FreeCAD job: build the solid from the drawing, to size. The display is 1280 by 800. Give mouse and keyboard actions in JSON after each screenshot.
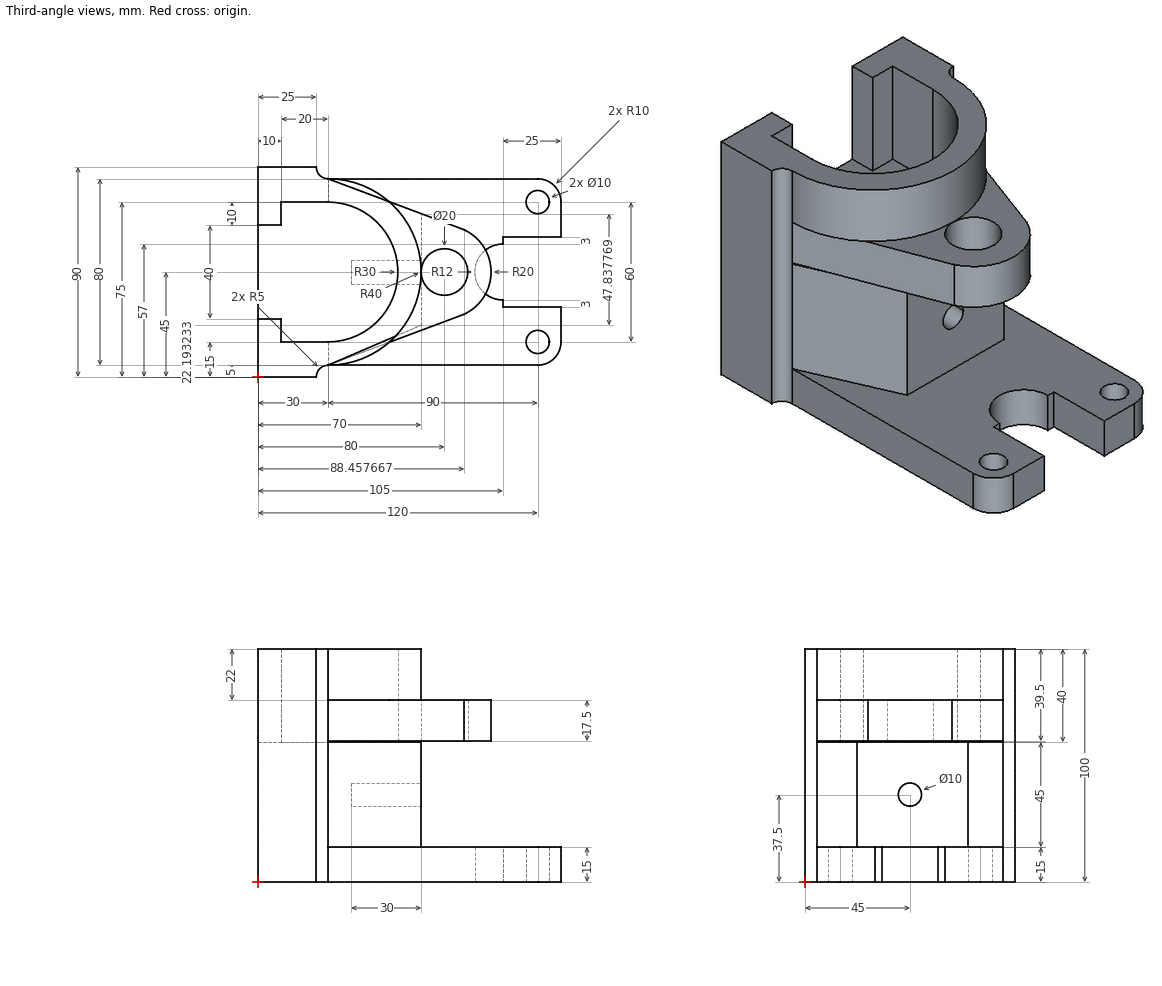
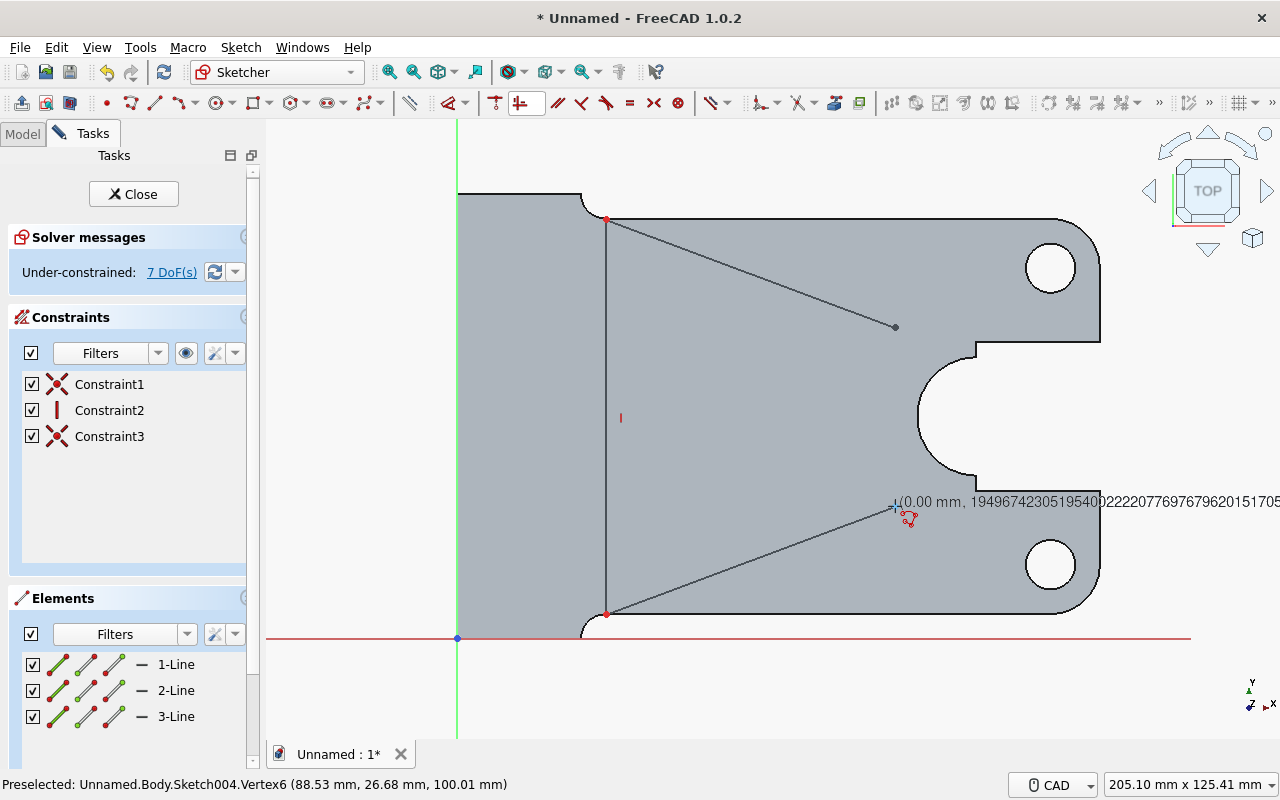
{"action": "left_click", "coordinate": [180, 104]}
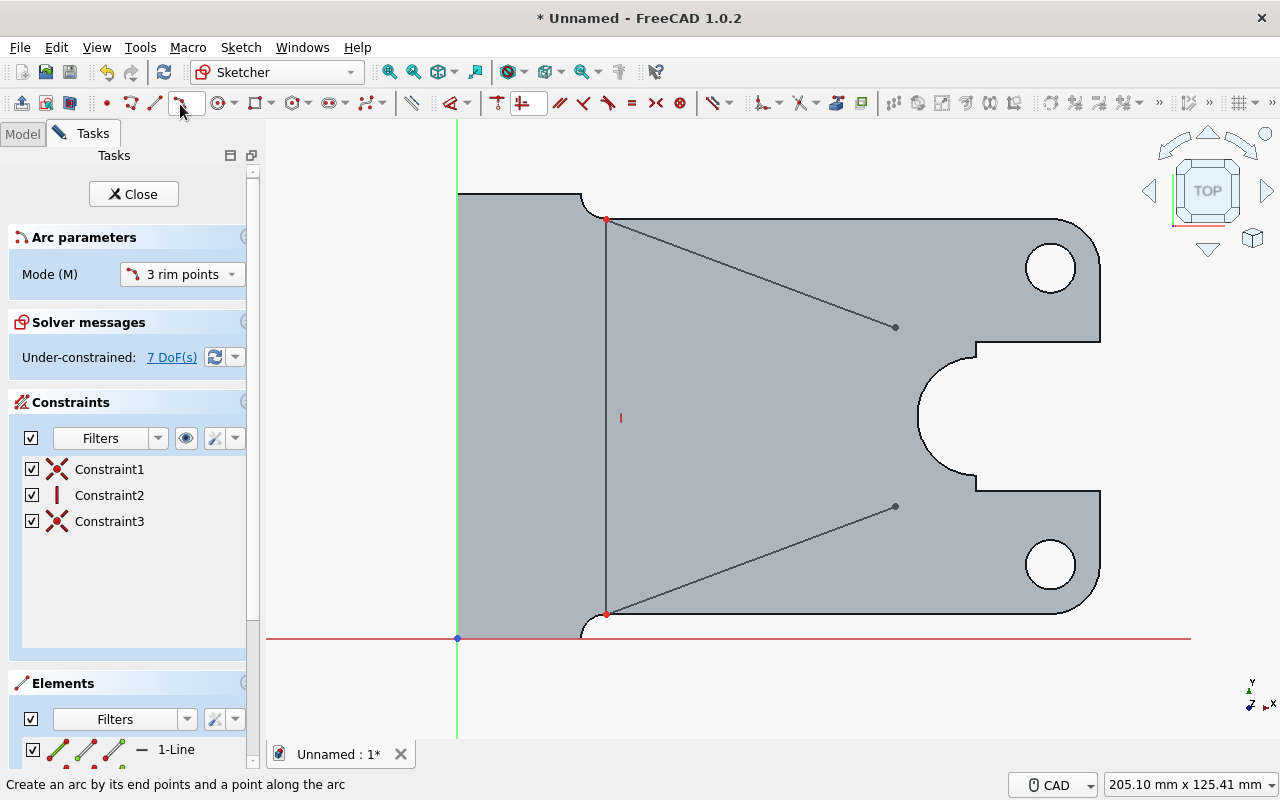
{"action": "left_click", "coordinate": [895, 507]}
{"action": "left_click", "coordinate": [895, 328]}
{"action": "left_click", "coordinate": [952, 416]}
{"action": "key", "text": "Escape"}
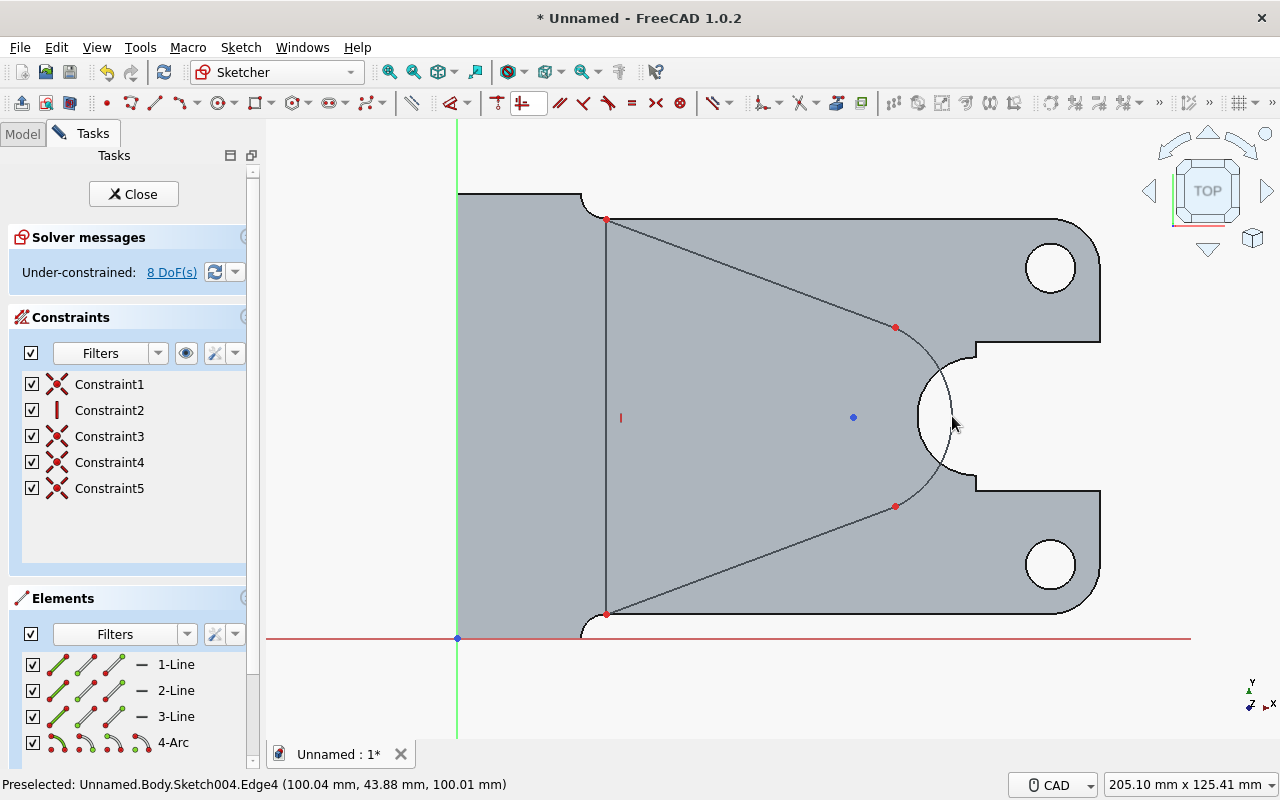
{"action": "key", "text": "d"}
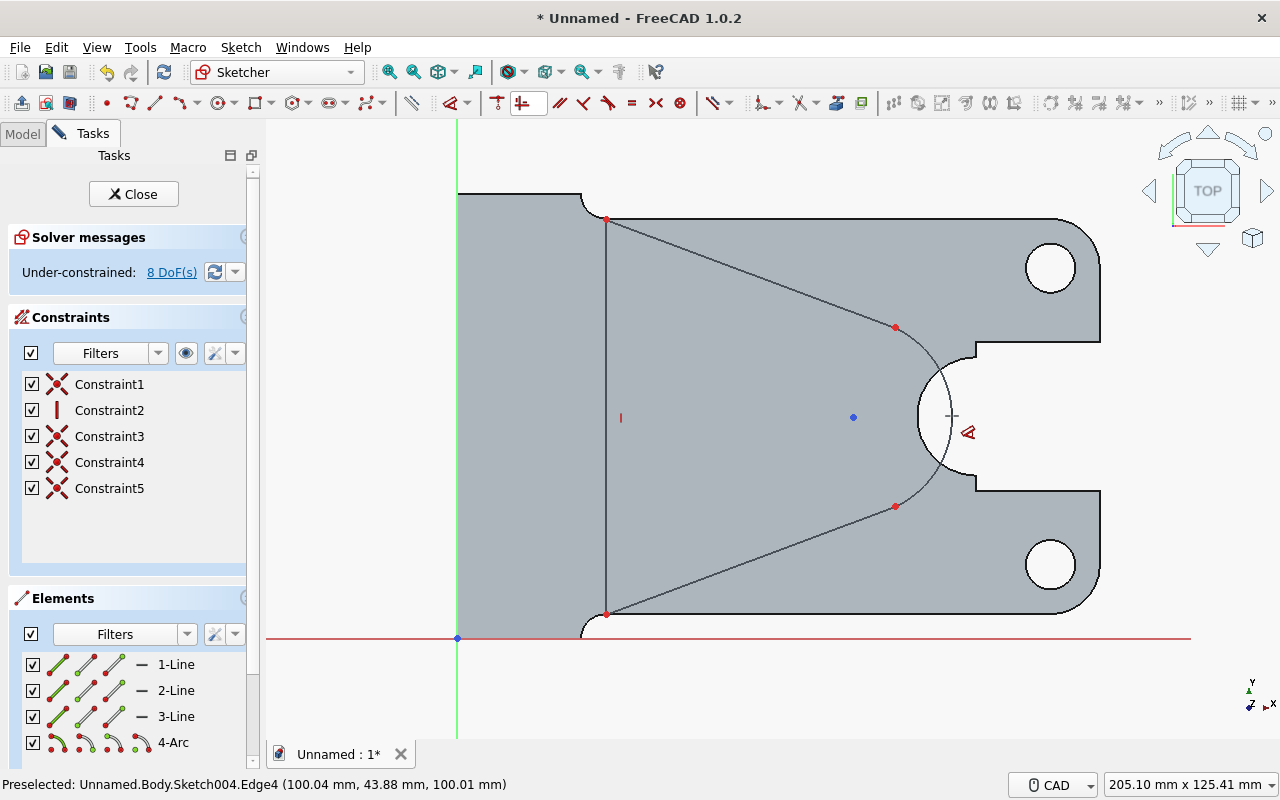
{"action": "left_click", "coordinate": [942, 461]}
{"action": "left_click", "coordinate": [971, 475]}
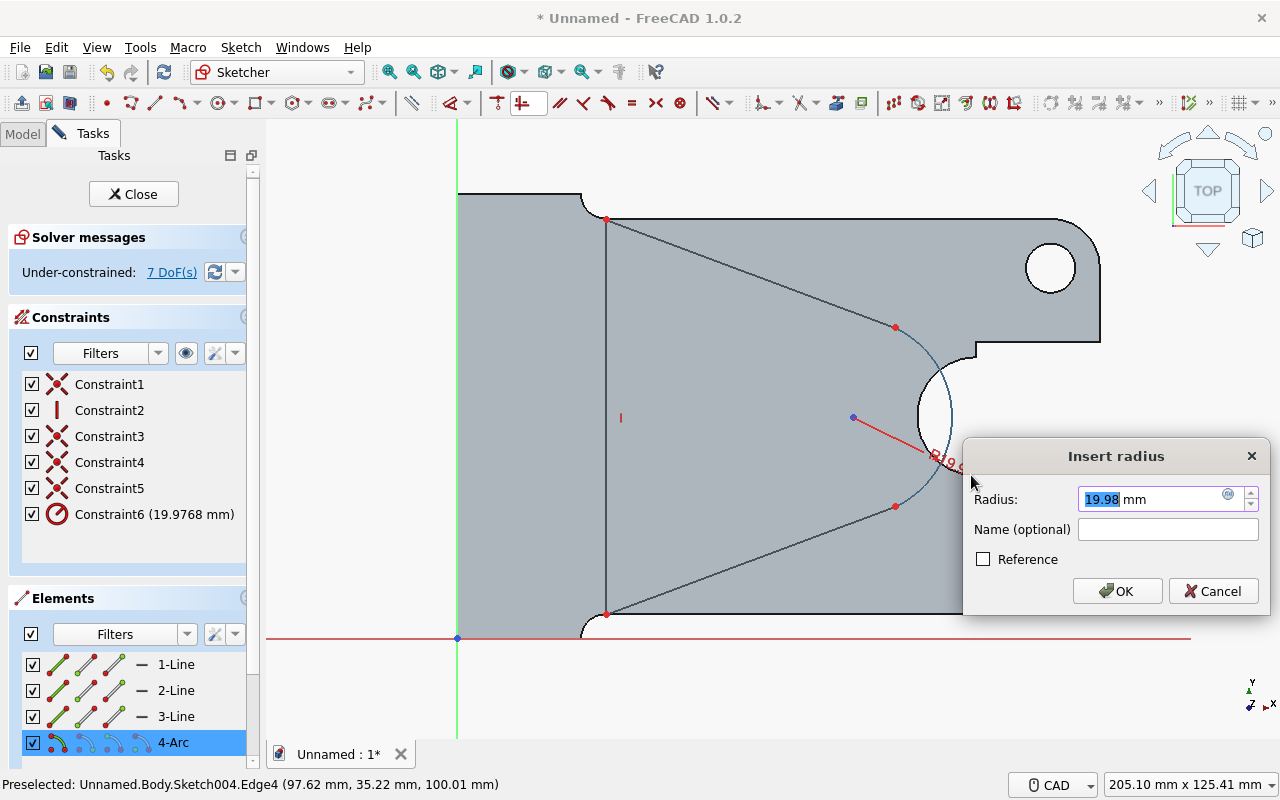
{"action": "type", "text": "20"}
{"action": "key", "text": "Return"}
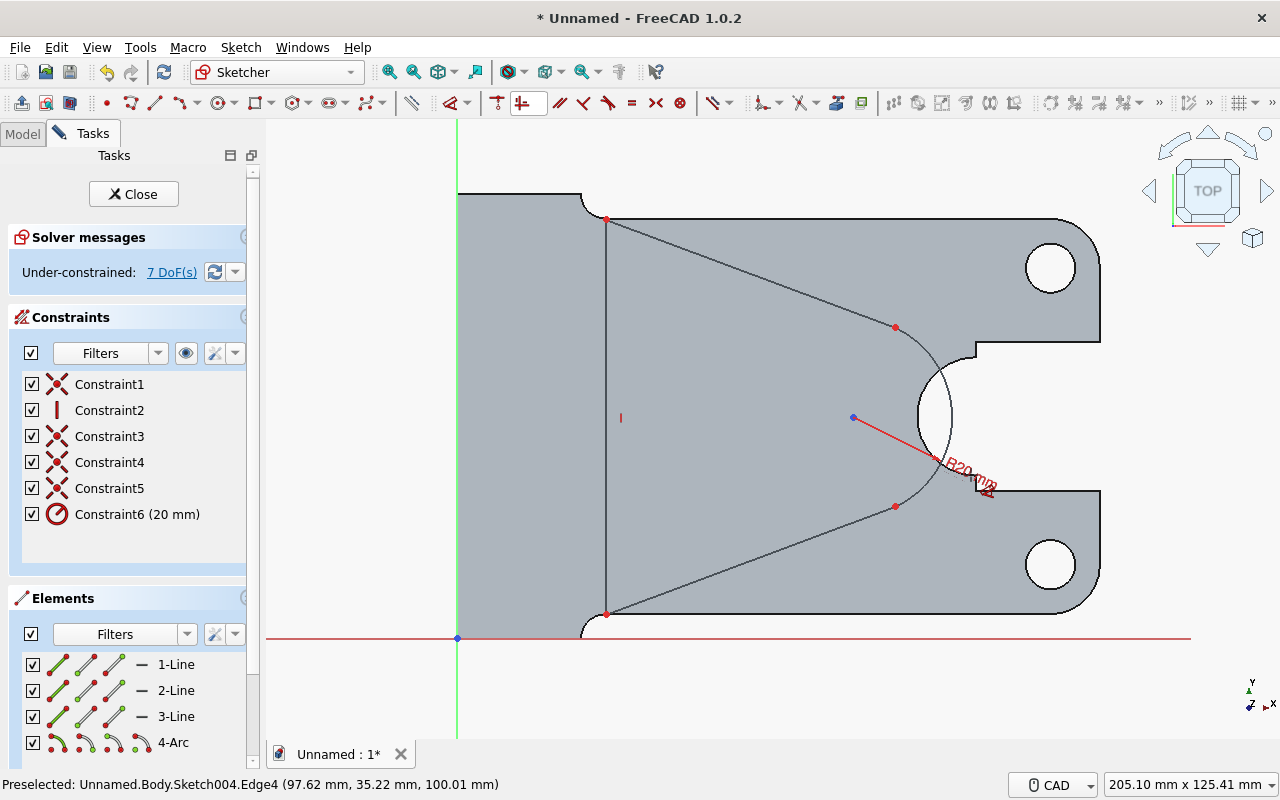
{"action": "left_click", "coordinate": [606, 339]}
{"action": "left_click", "coordinate": [572, 418]}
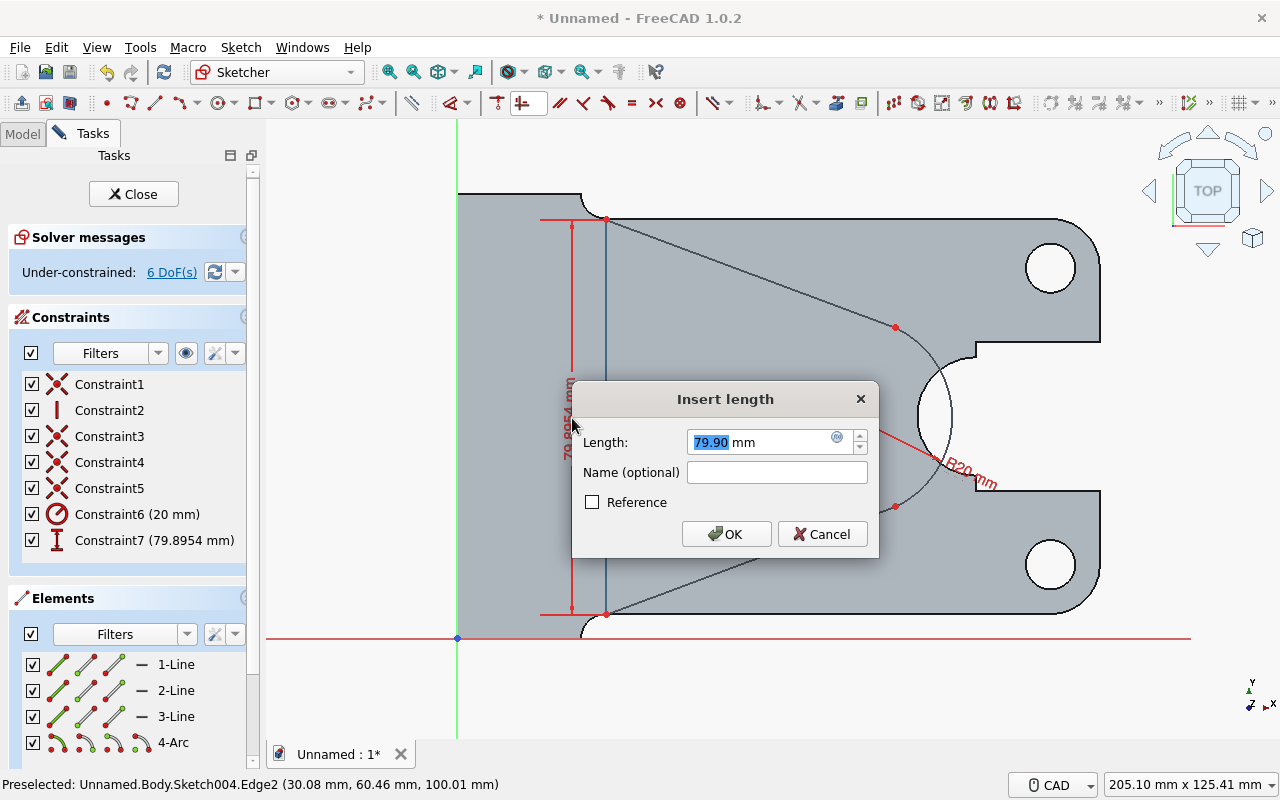
{"action": "type", "text": "80"}
{"action": "key", "text": "Return"}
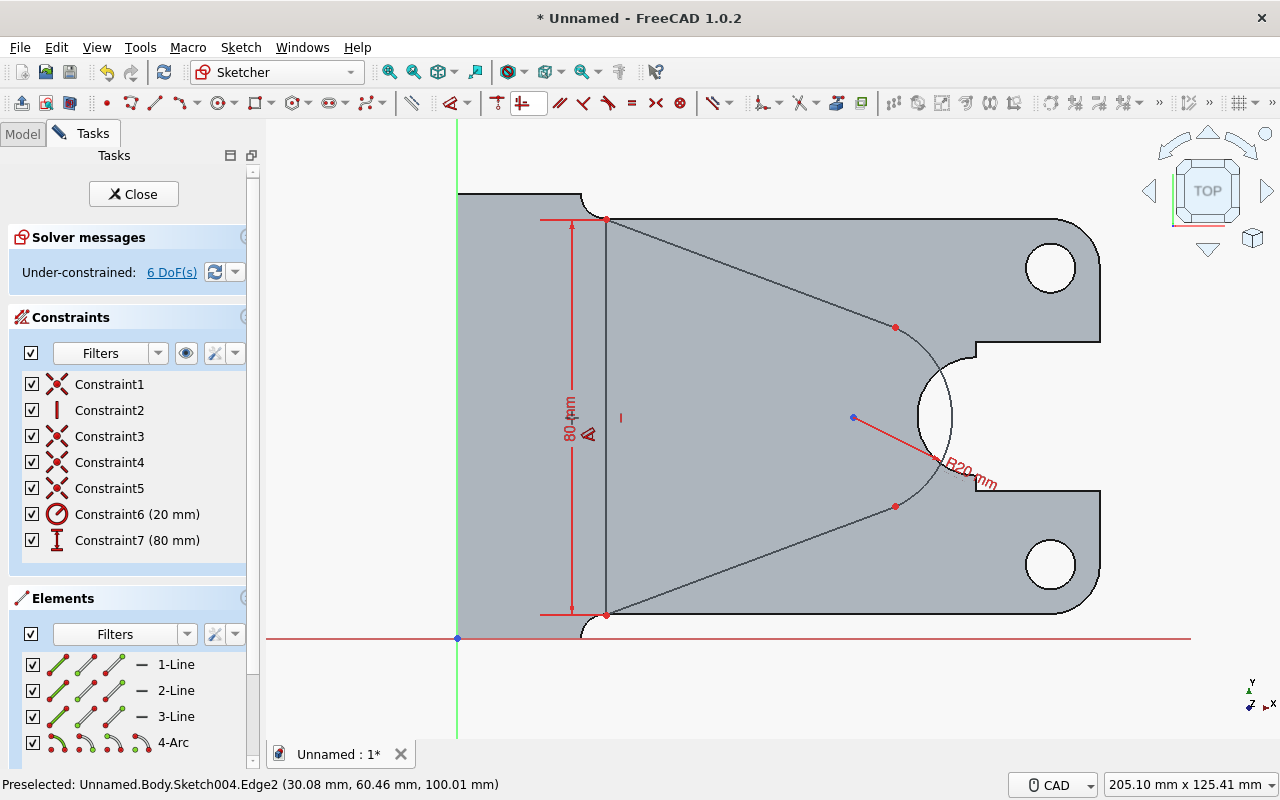
{"action": "scroll", "coordinate": [606, 615], "scroll_direction": "up", "scroll_amount": 3}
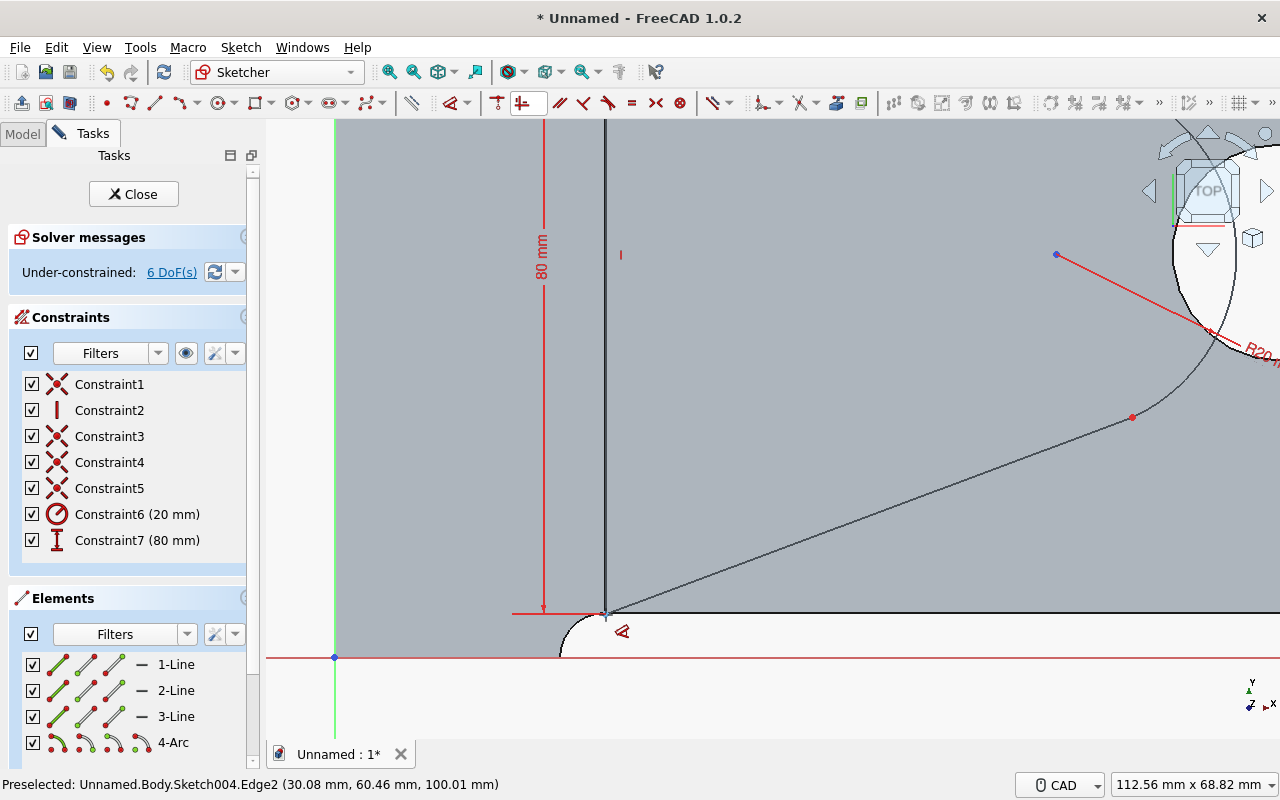
{"action": "left_click", "coordinate": [606, 614]}
{"action": "left_click", "coordinate": [301, 636]}